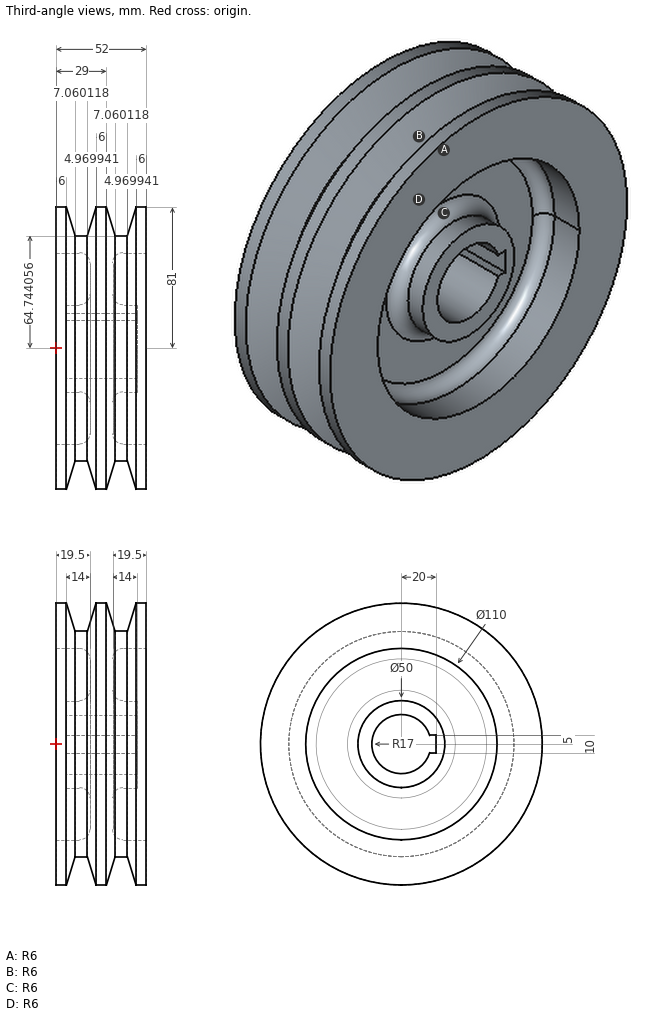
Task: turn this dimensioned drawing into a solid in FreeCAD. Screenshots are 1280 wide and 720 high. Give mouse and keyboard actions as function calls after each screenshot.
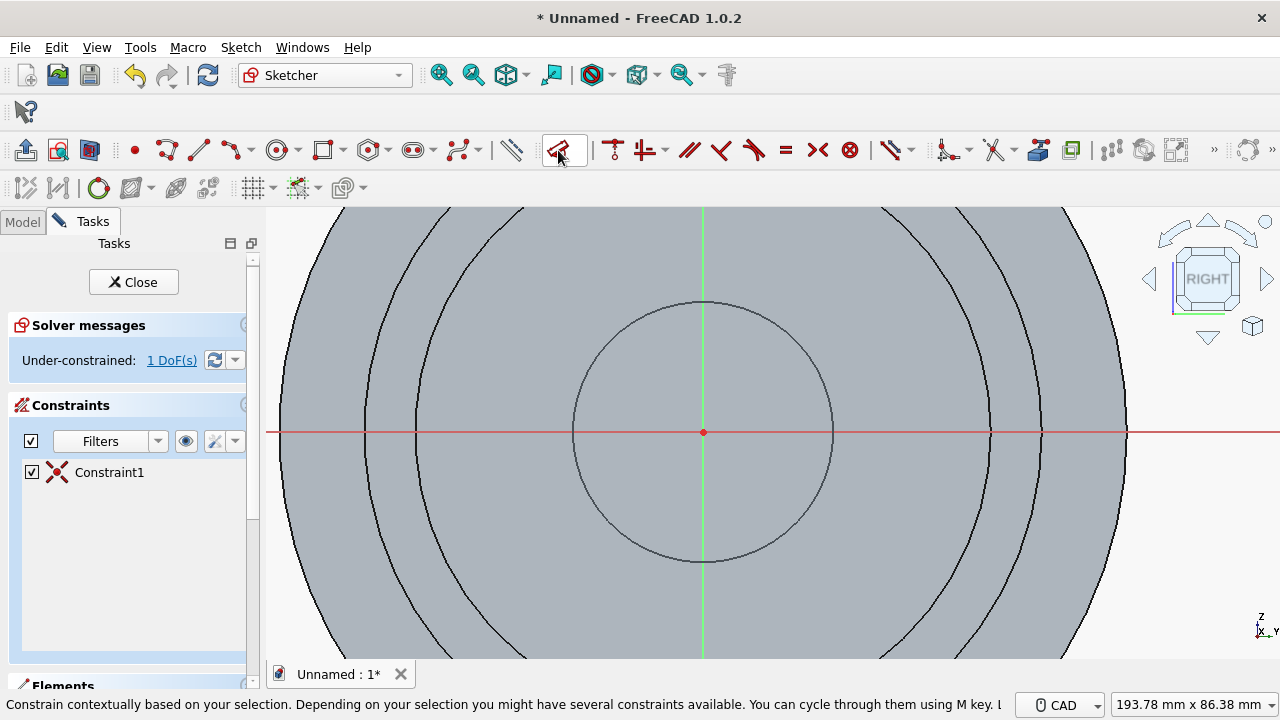
click(795, 340)
click(818, 317)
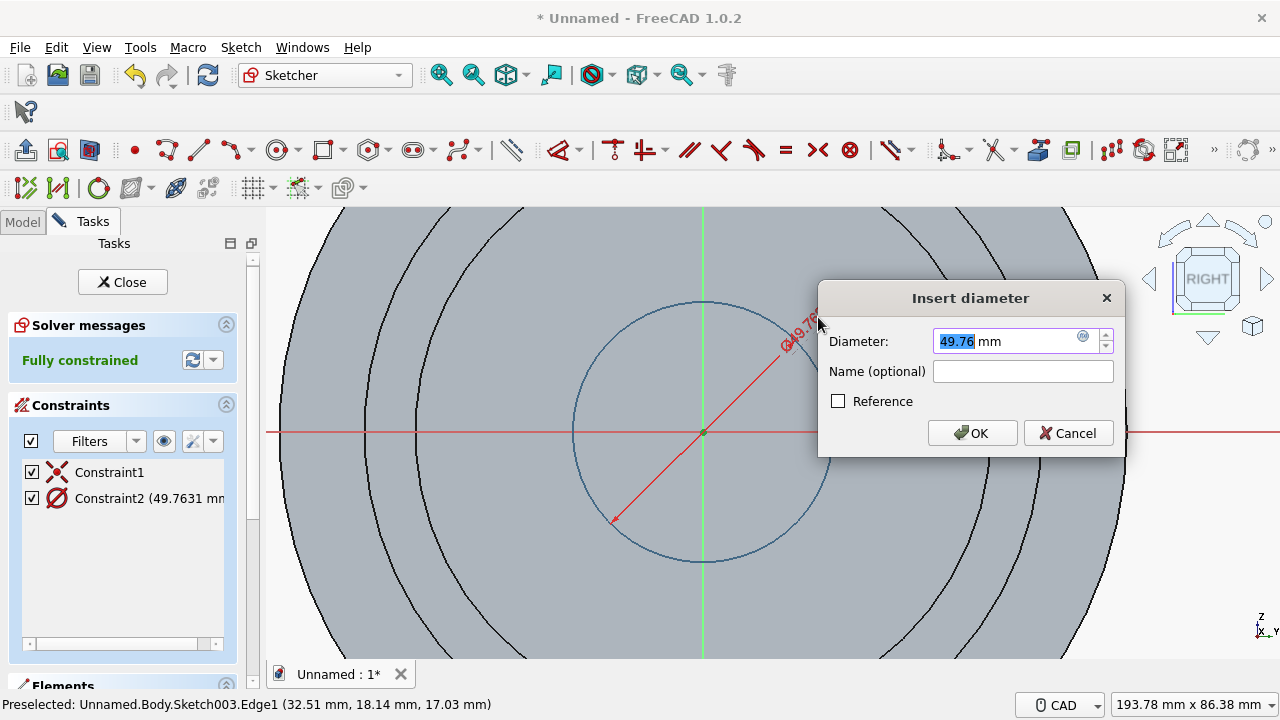
text(50)
key(Return)
key(Escape)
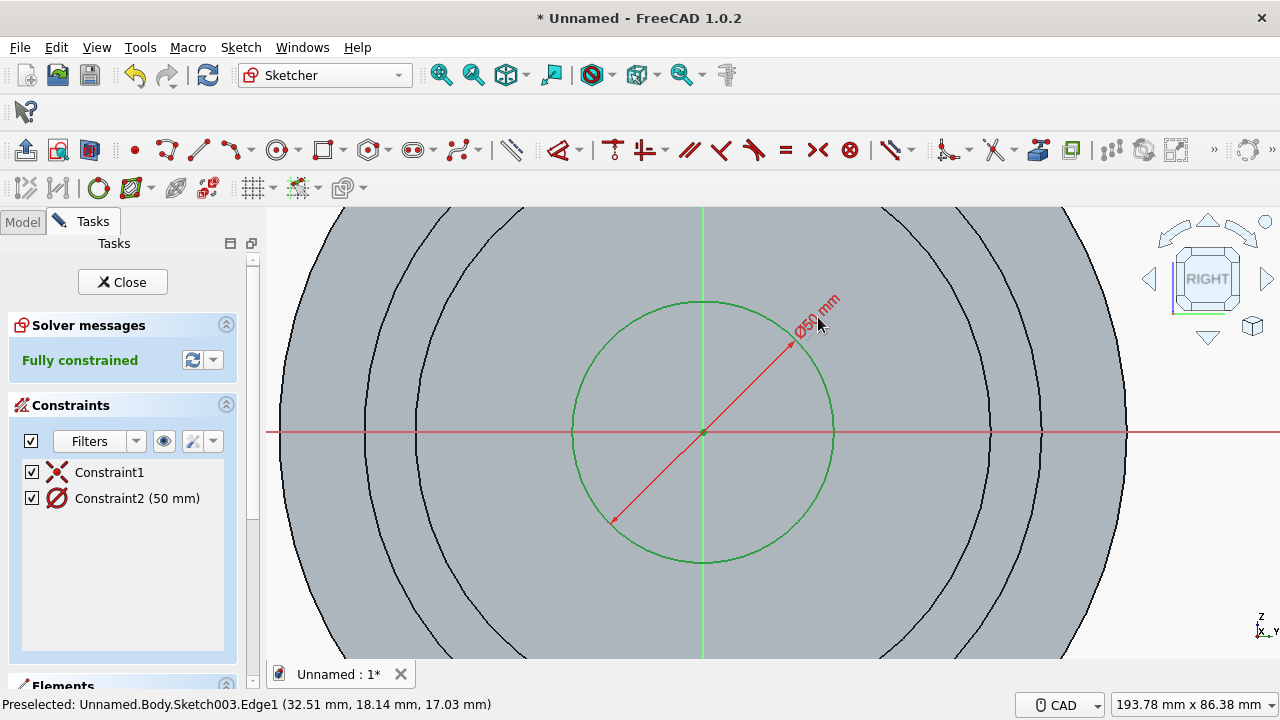
click(123, 282)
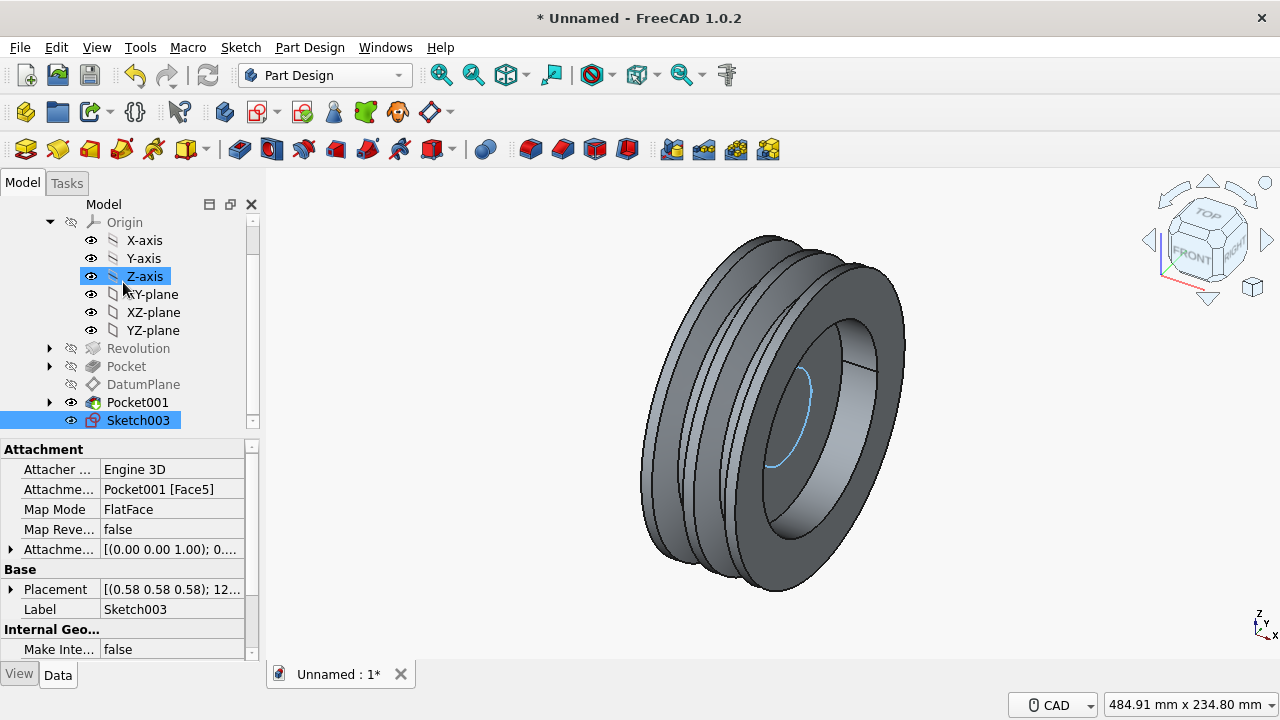
click(26, 150)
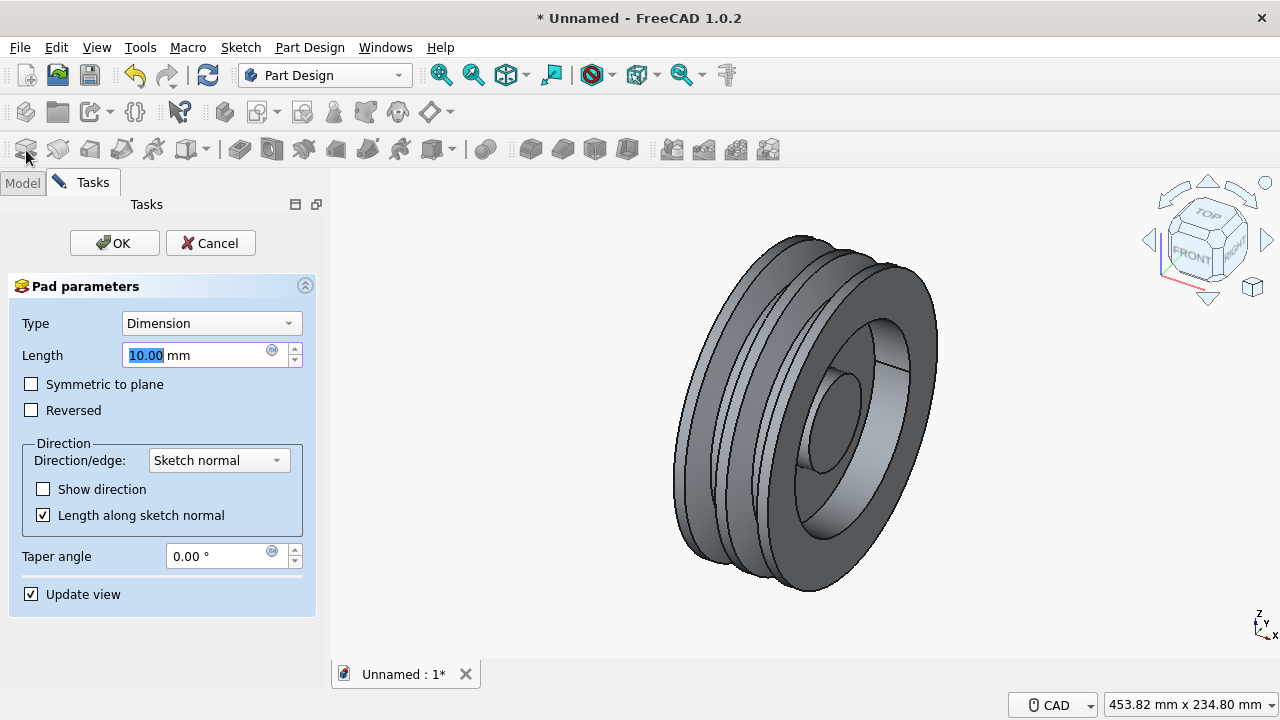
text(14)
key(Tab)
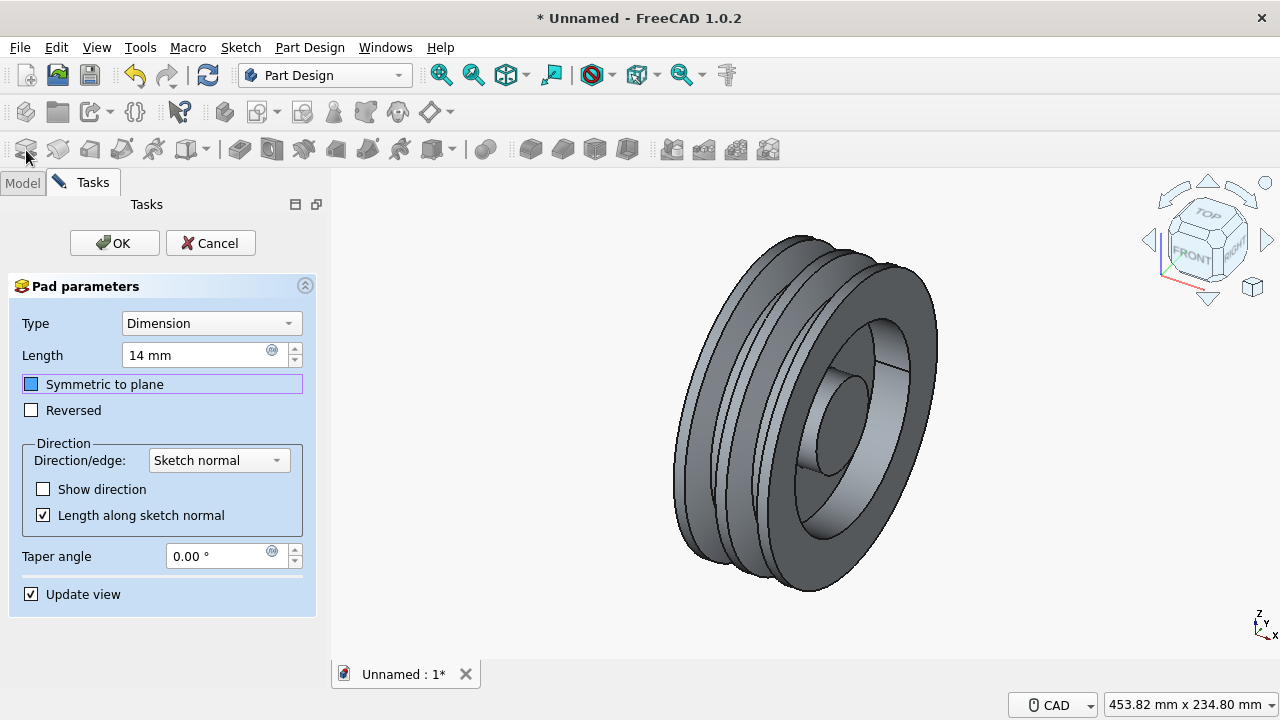
click(115, 243)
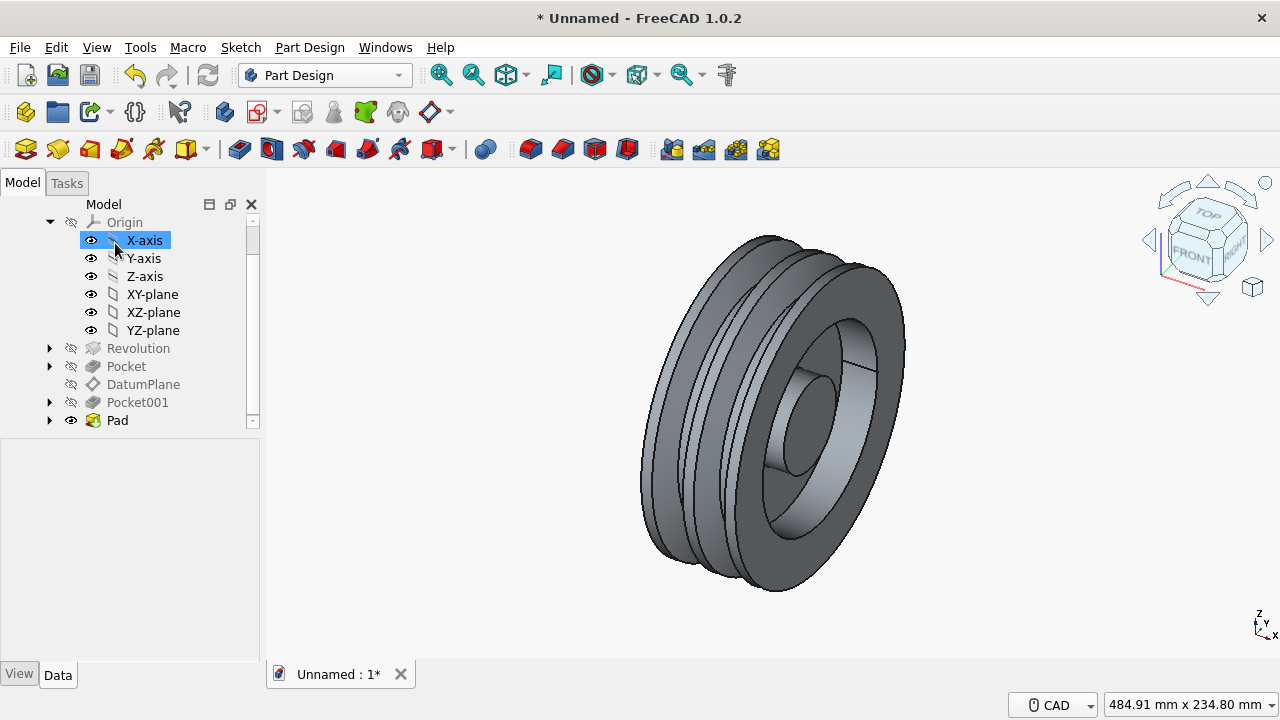
click(136, 330)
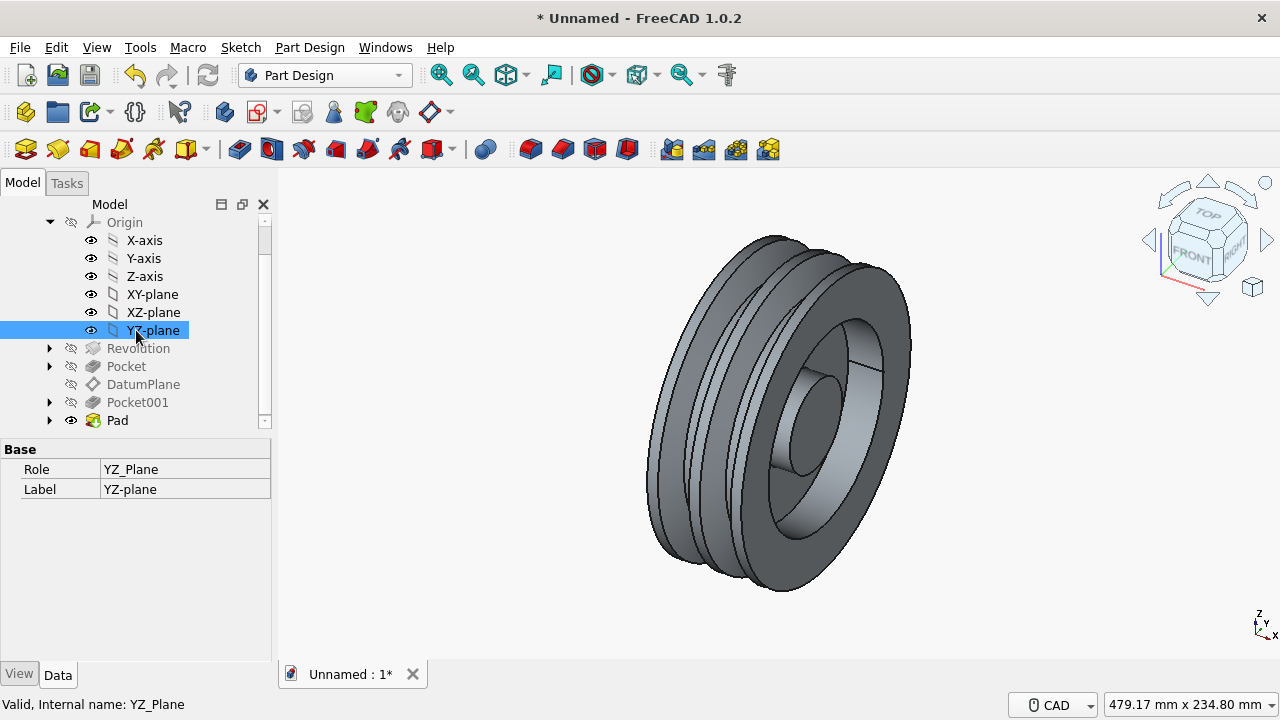
click(430, 112)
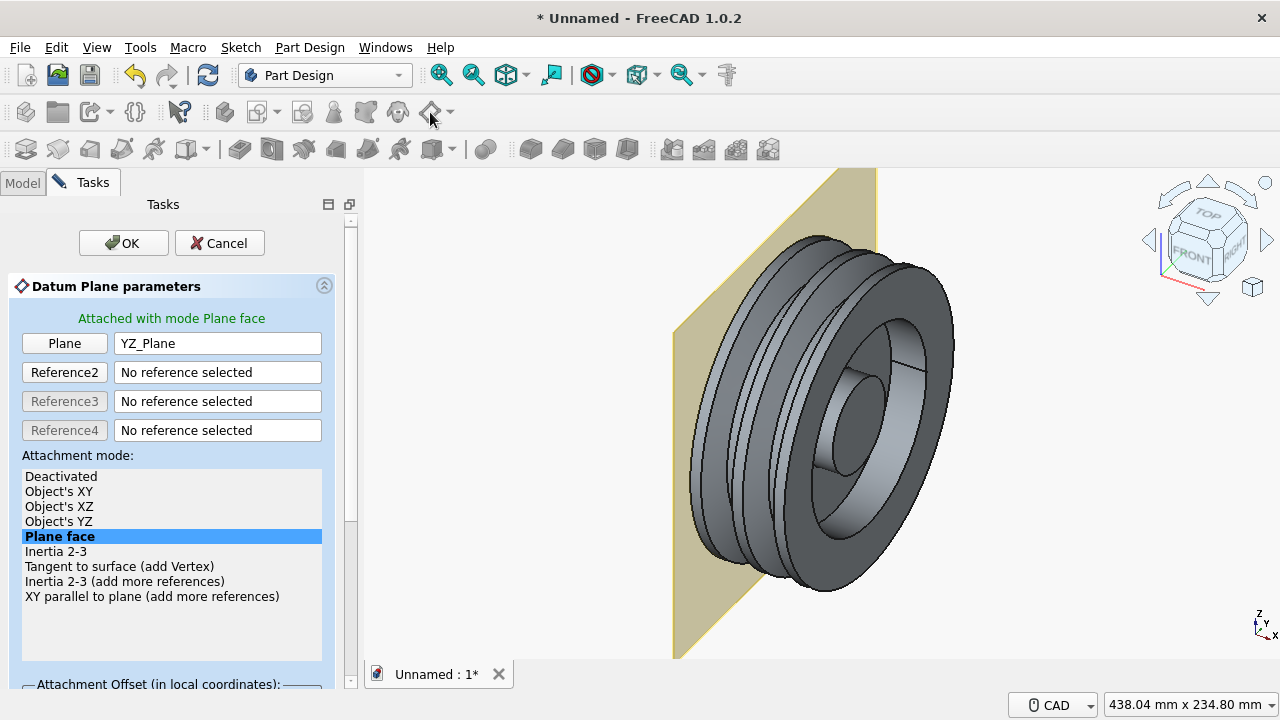
scroll(351, 451, down, 3)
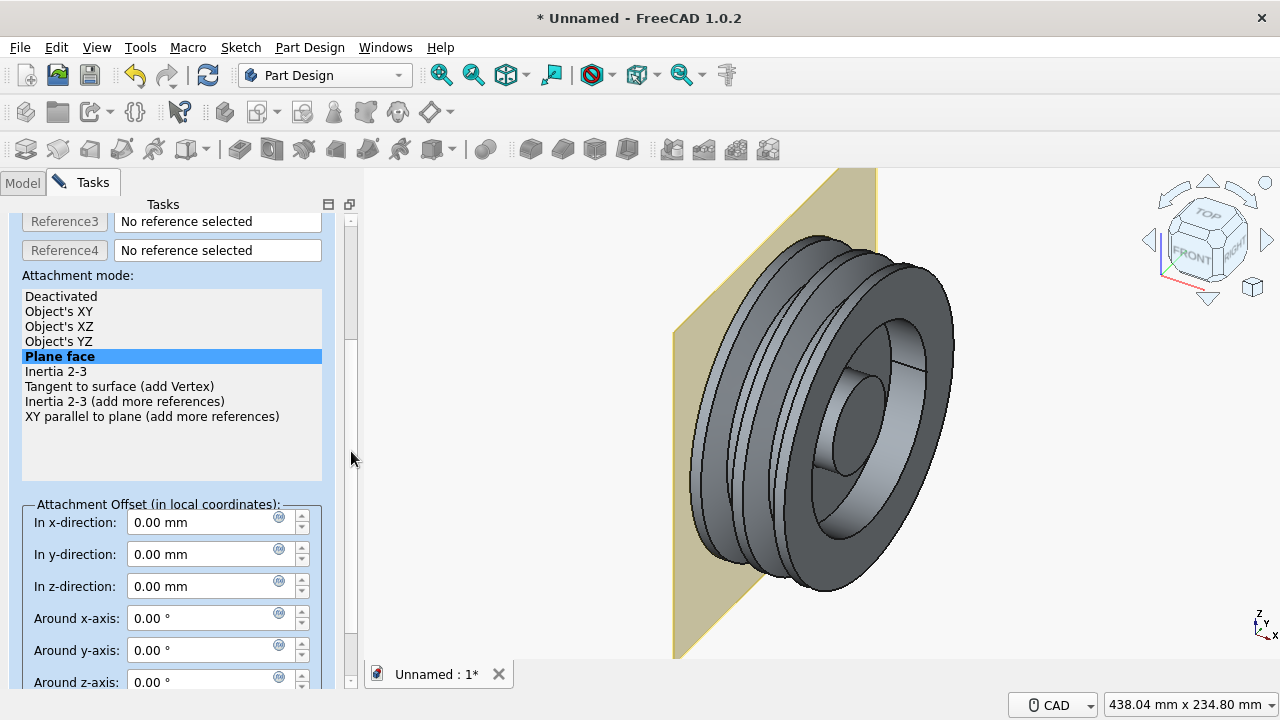
triple_click(210, 586)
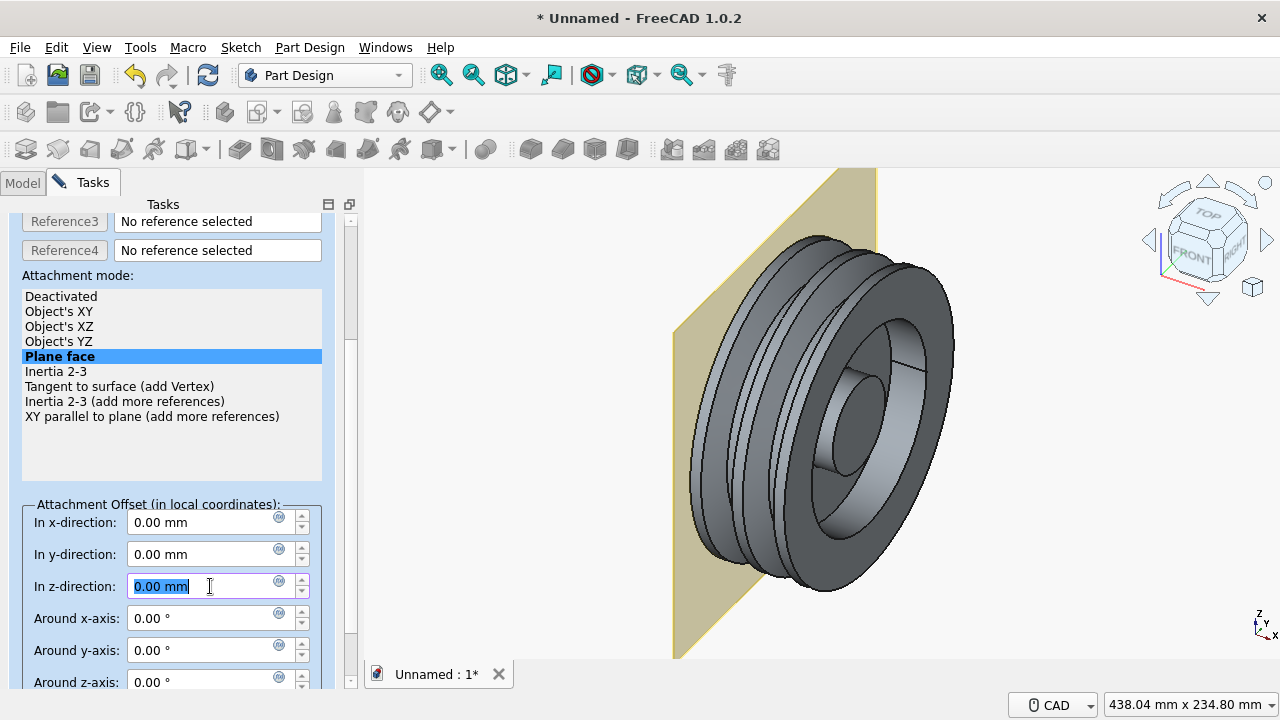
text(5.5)
key(Tab)